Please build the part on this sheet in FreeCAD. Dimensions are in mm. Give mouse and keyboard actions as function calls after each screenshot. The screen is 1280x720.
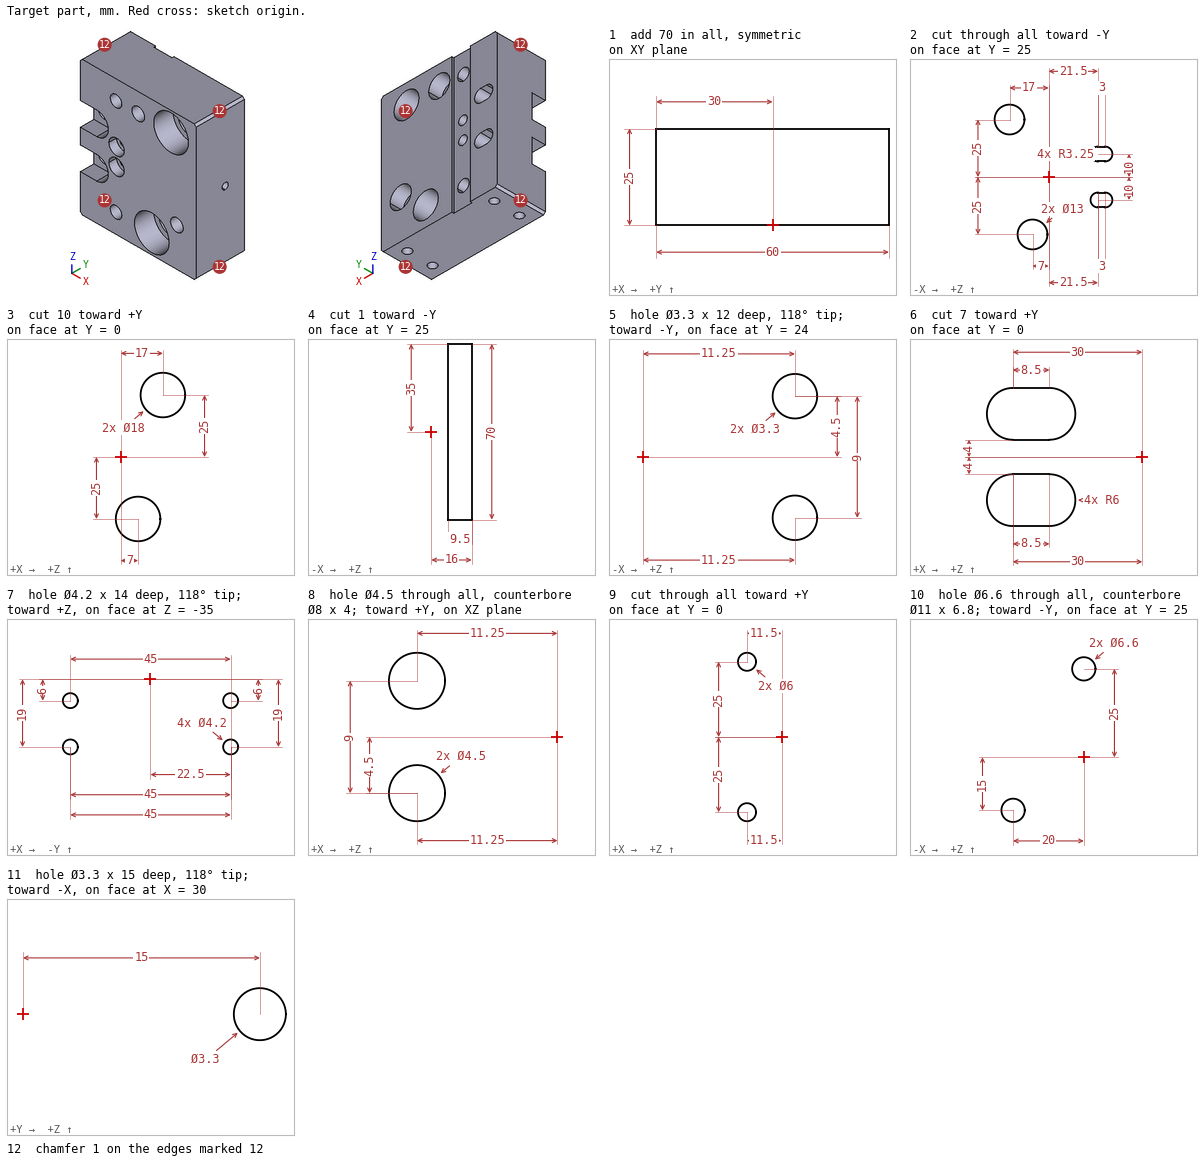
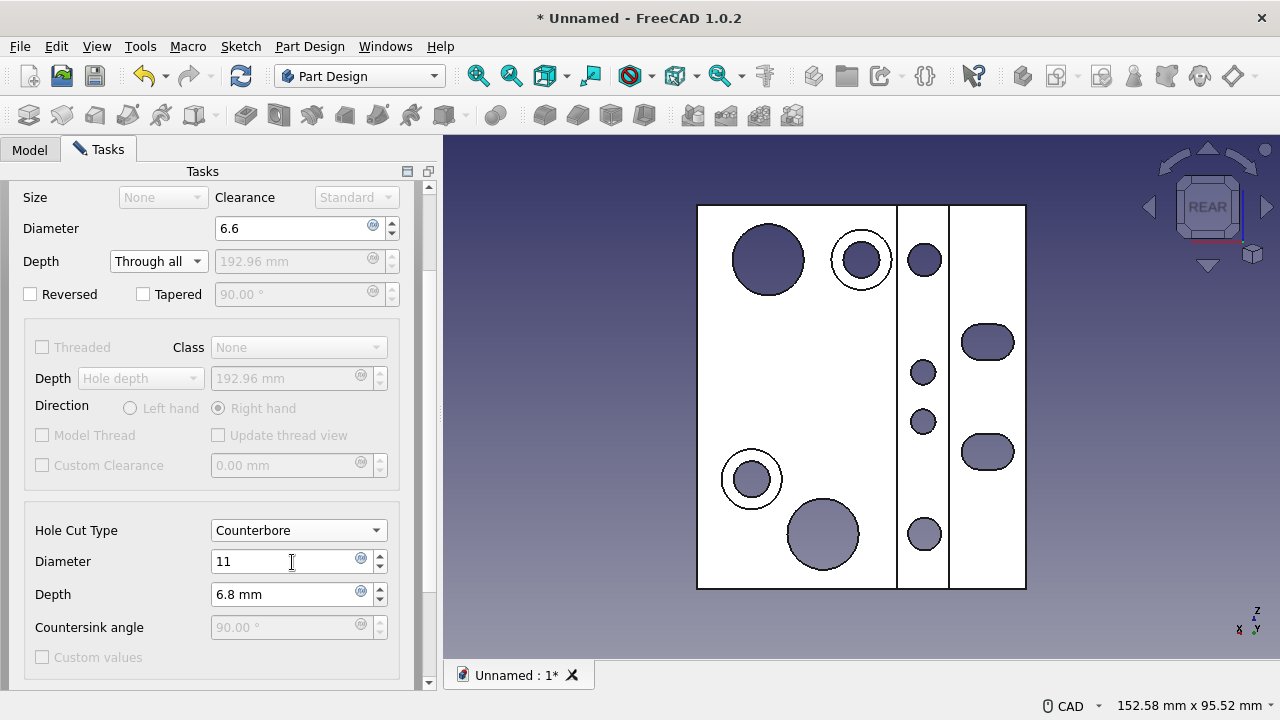
scroll(429, 436, up, 3)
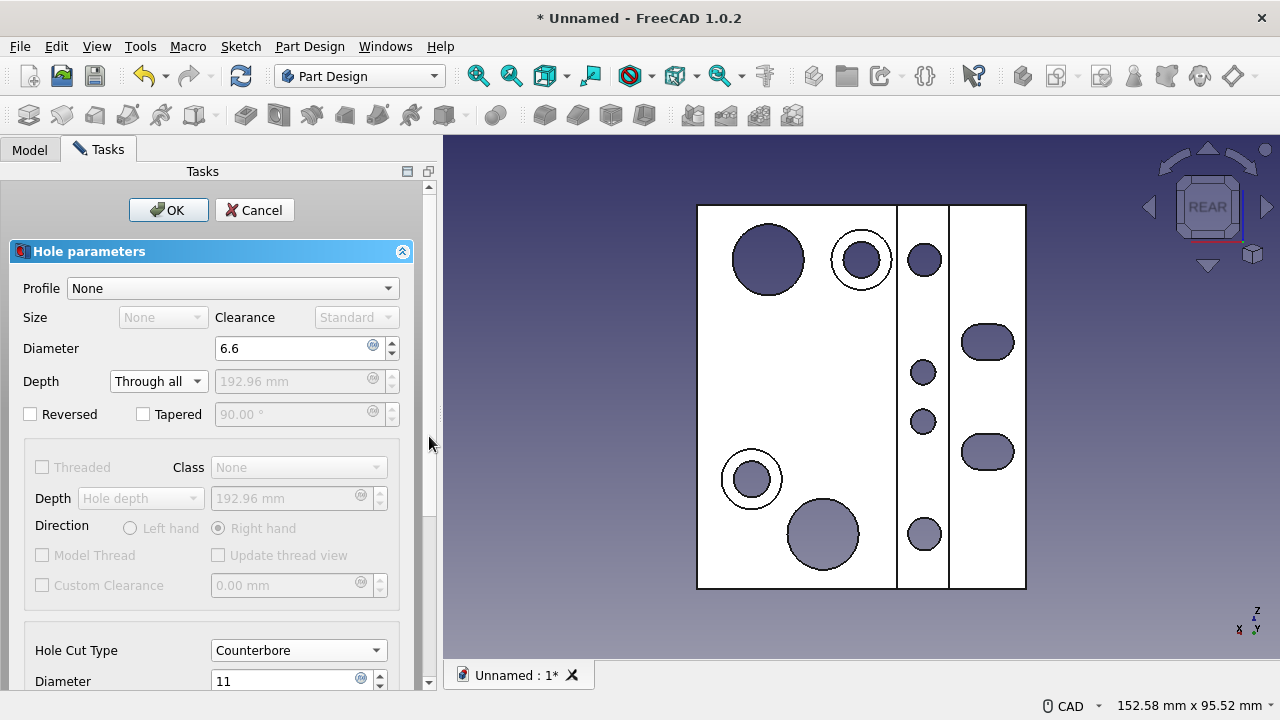
click(169, 210)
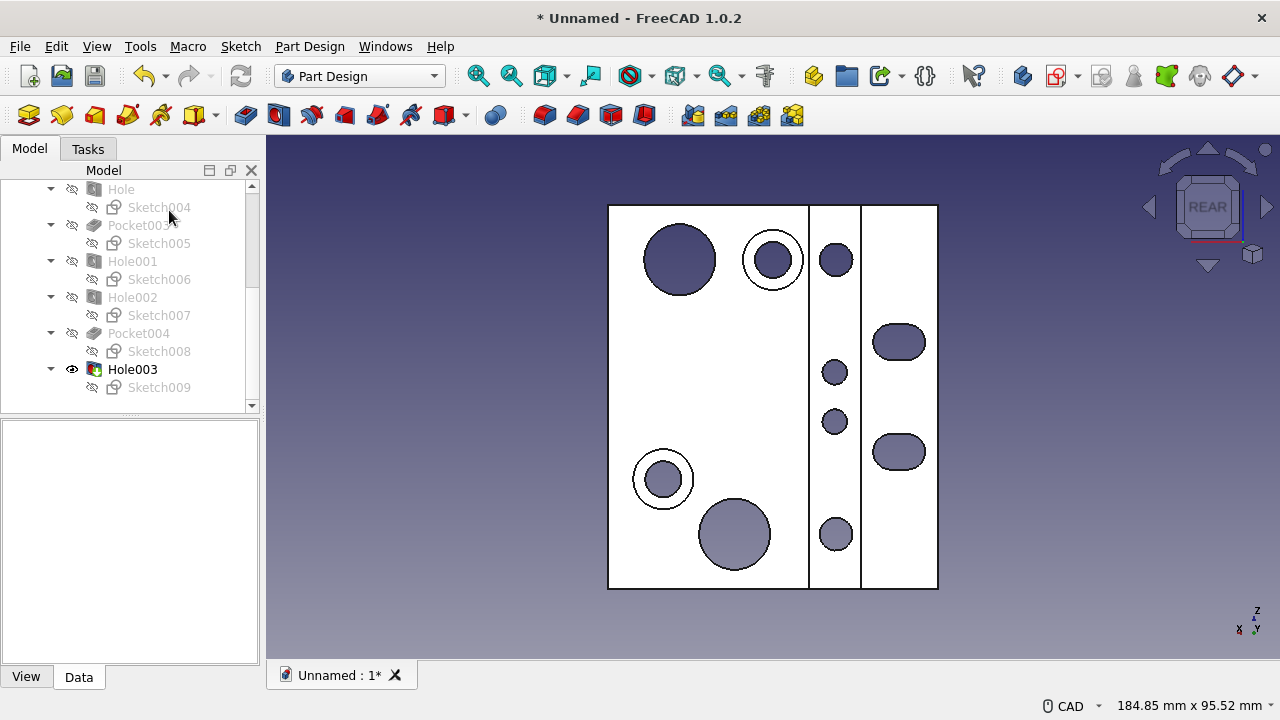
key(0)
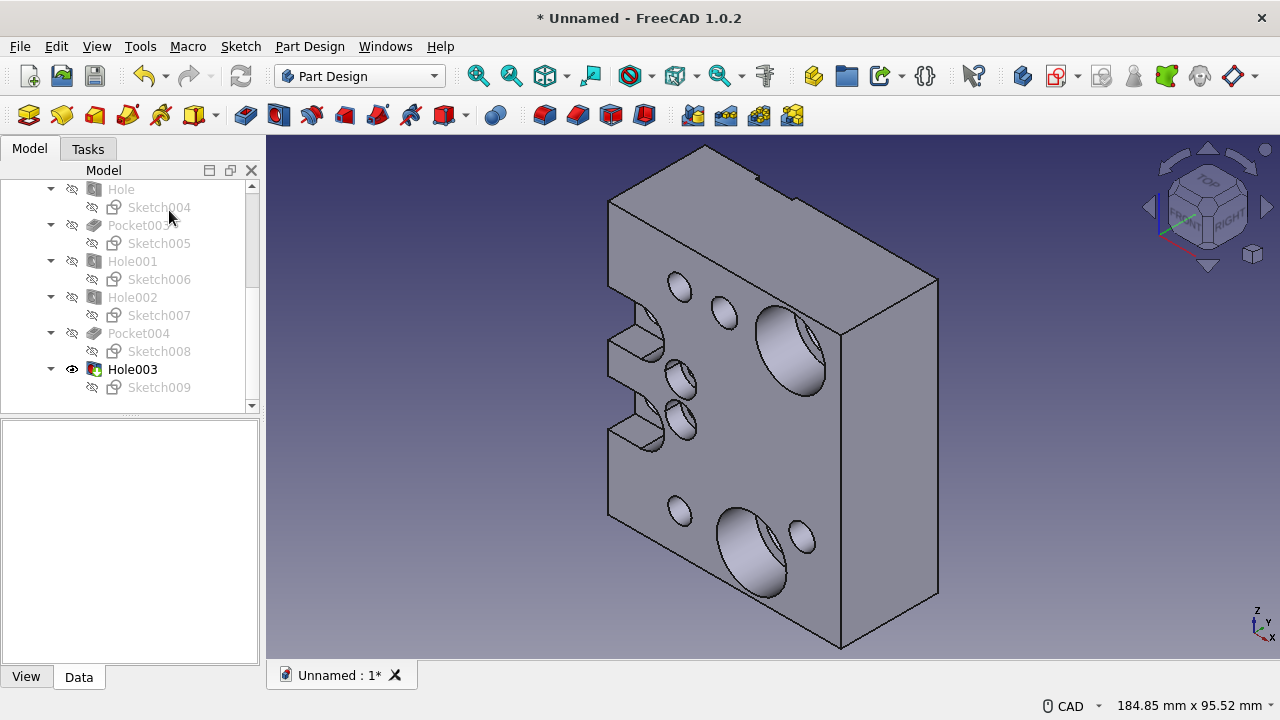
click(889, 374)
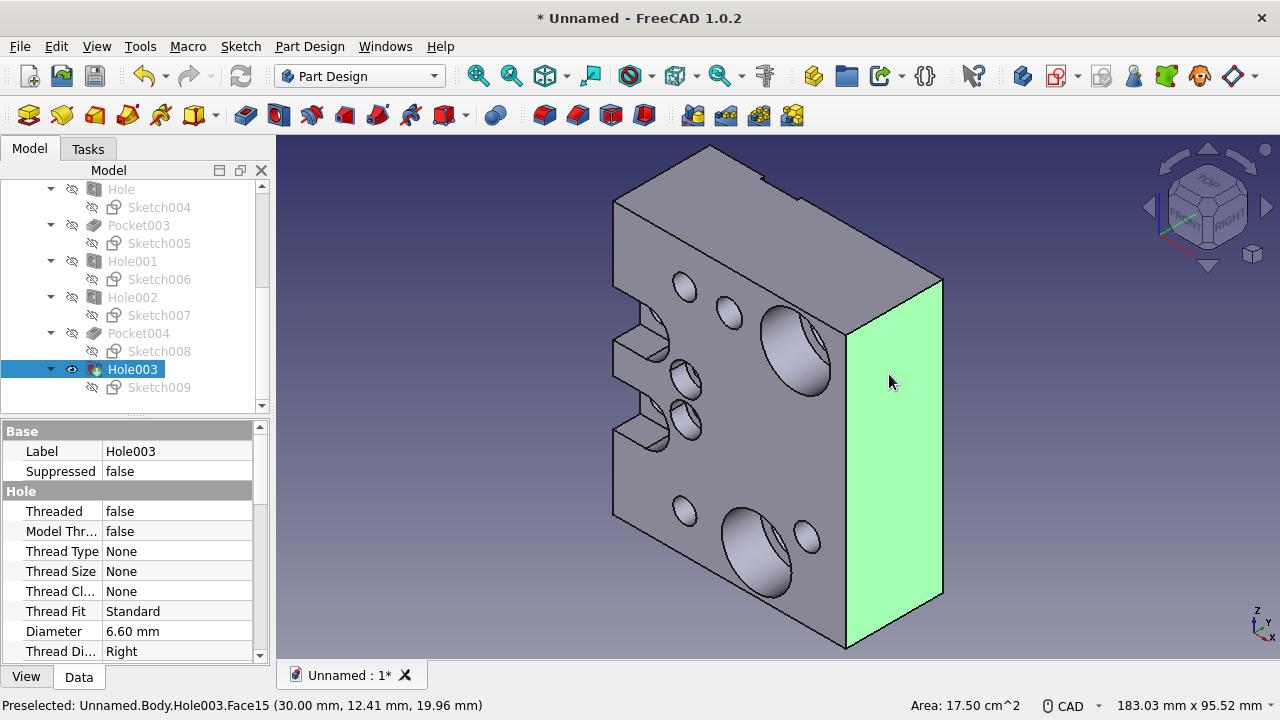
click(1056, 76)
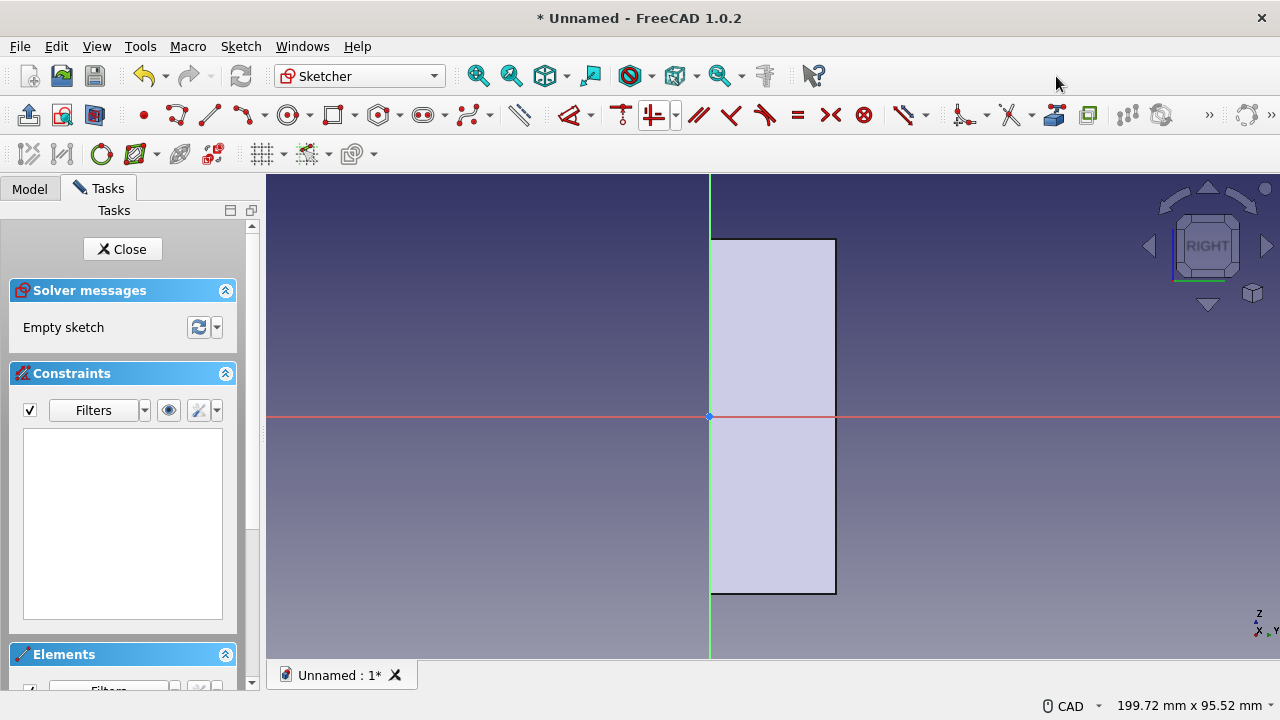
scroll(791, 416, up, 14)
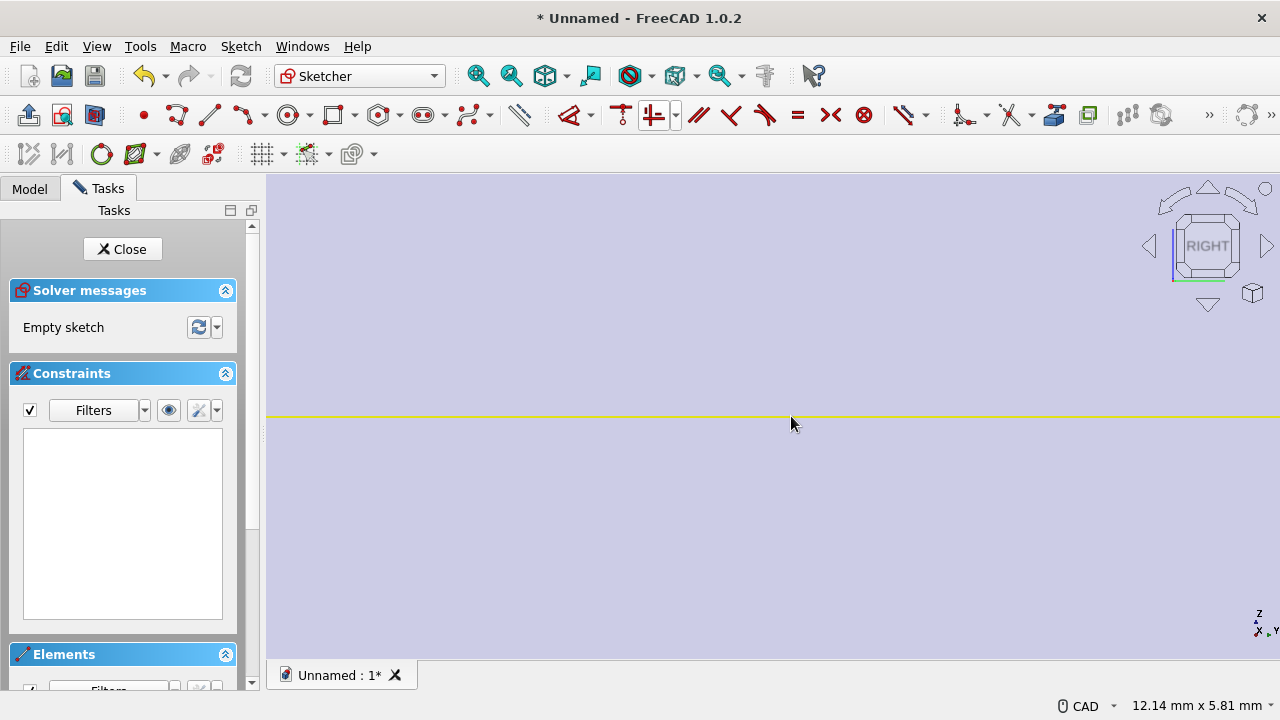
key(g)
key(c)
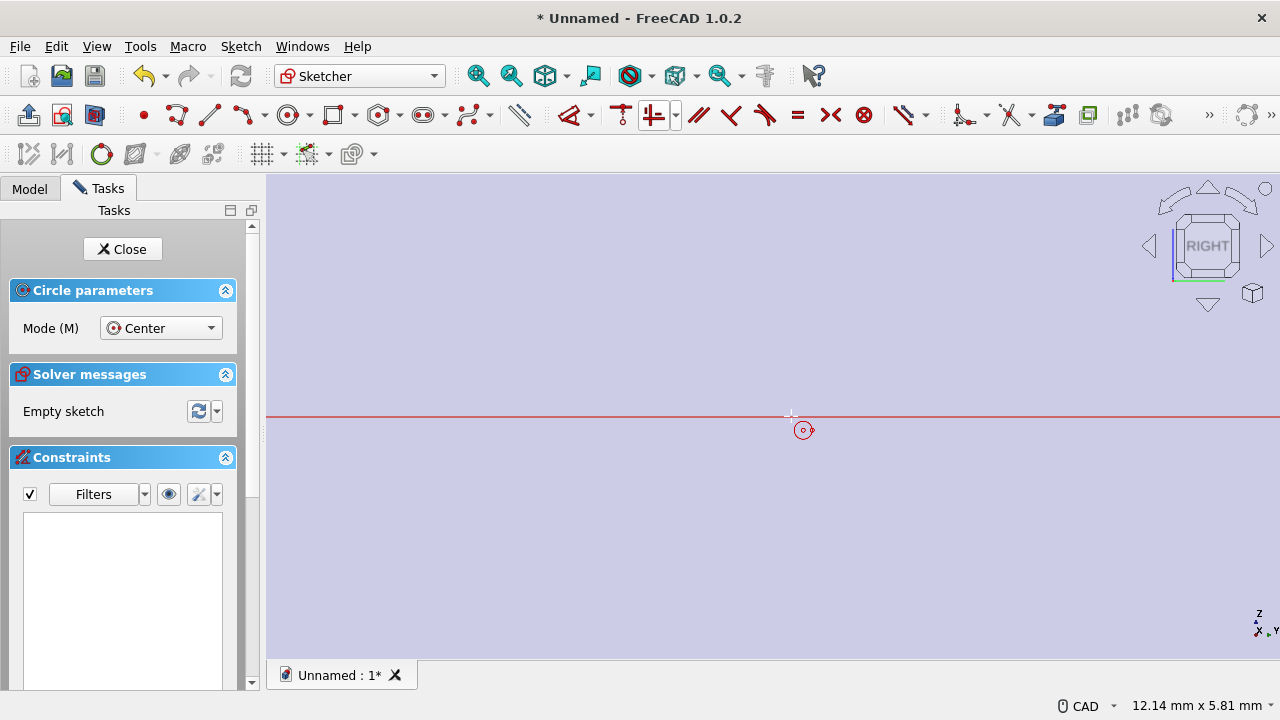
click(696, 416)
move(793, 319)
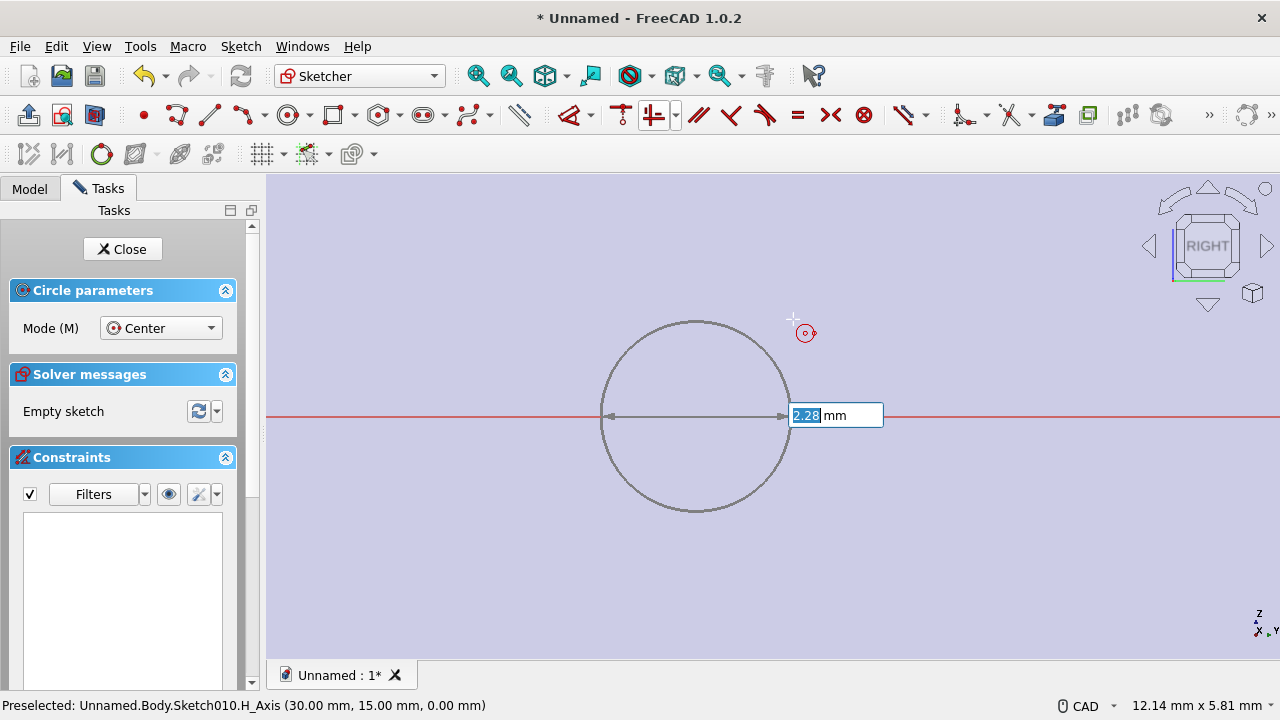
text(3.3)
key(Return)
key(Escape)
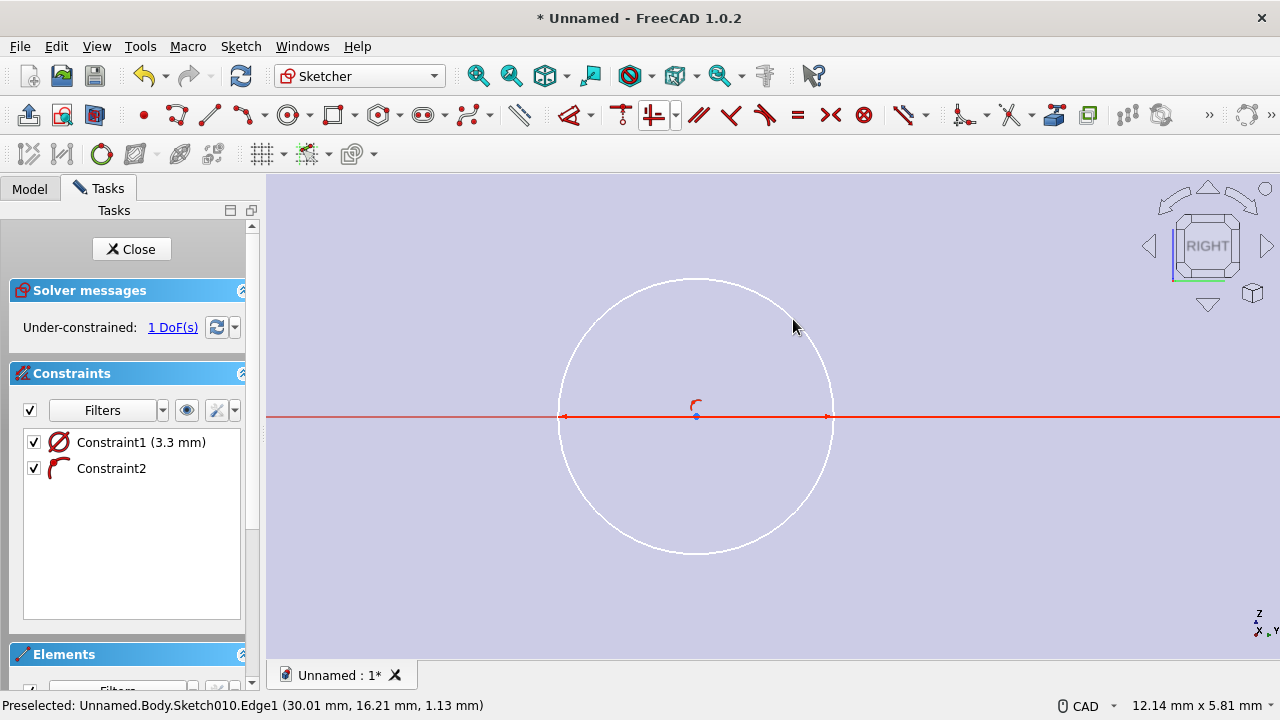
key(d)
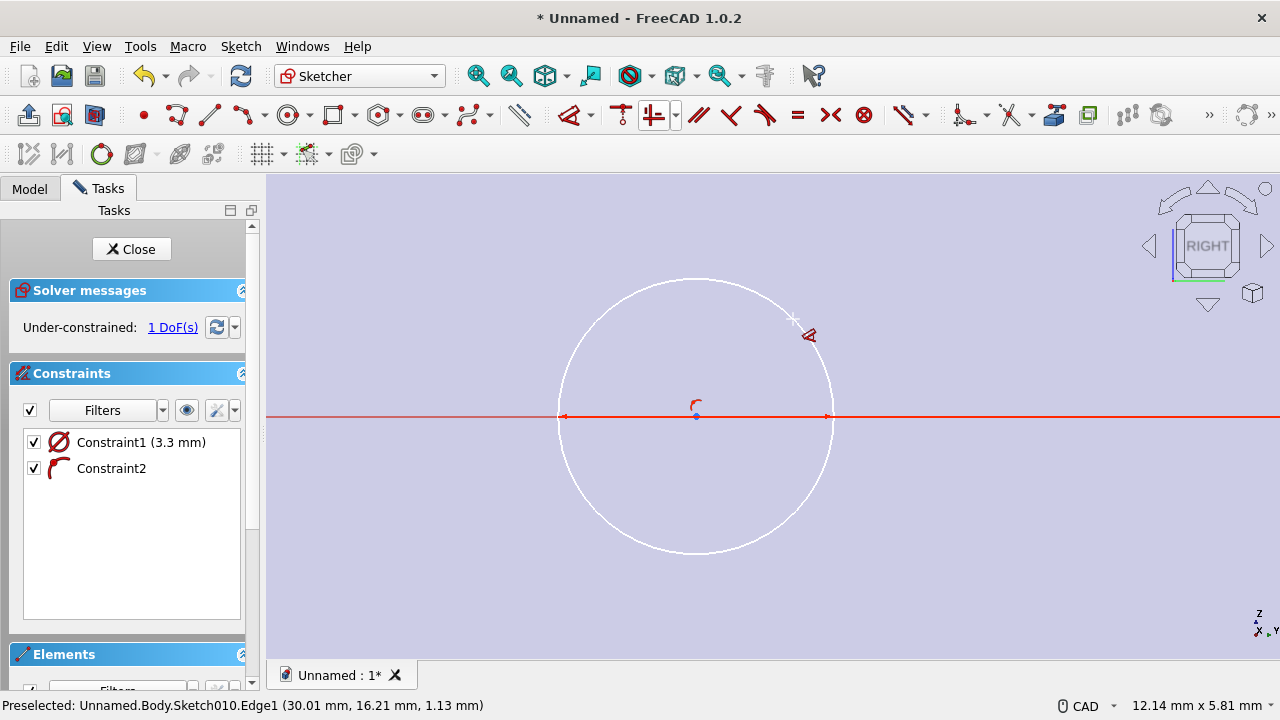
click(696, 416)
click(495, 450)